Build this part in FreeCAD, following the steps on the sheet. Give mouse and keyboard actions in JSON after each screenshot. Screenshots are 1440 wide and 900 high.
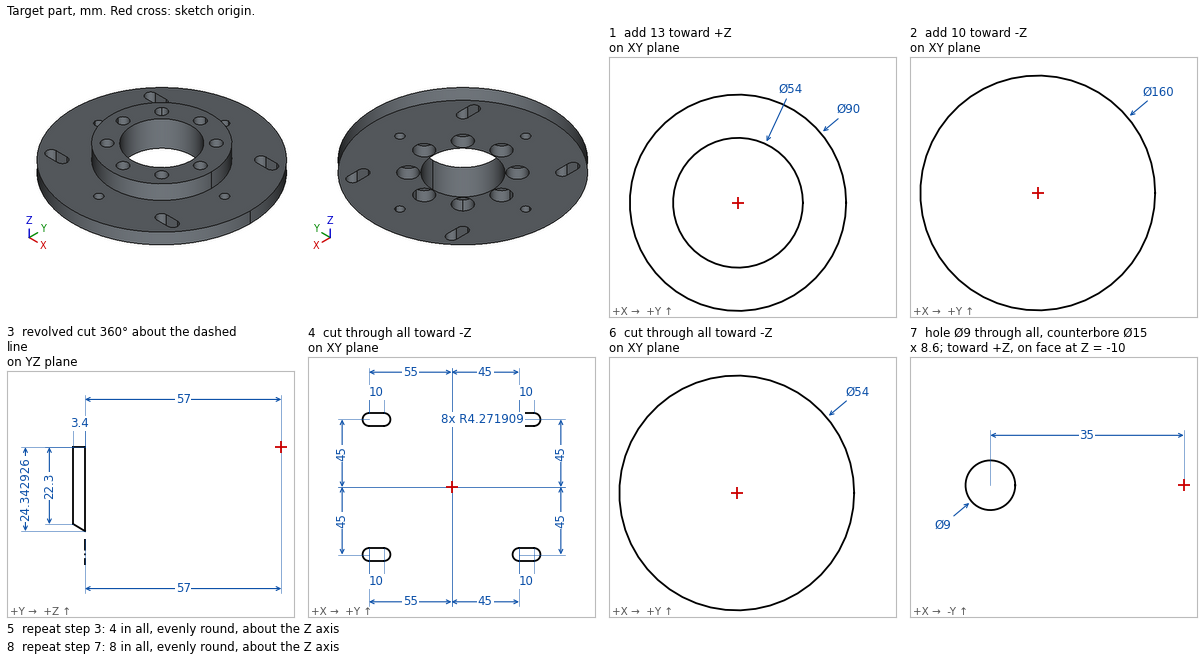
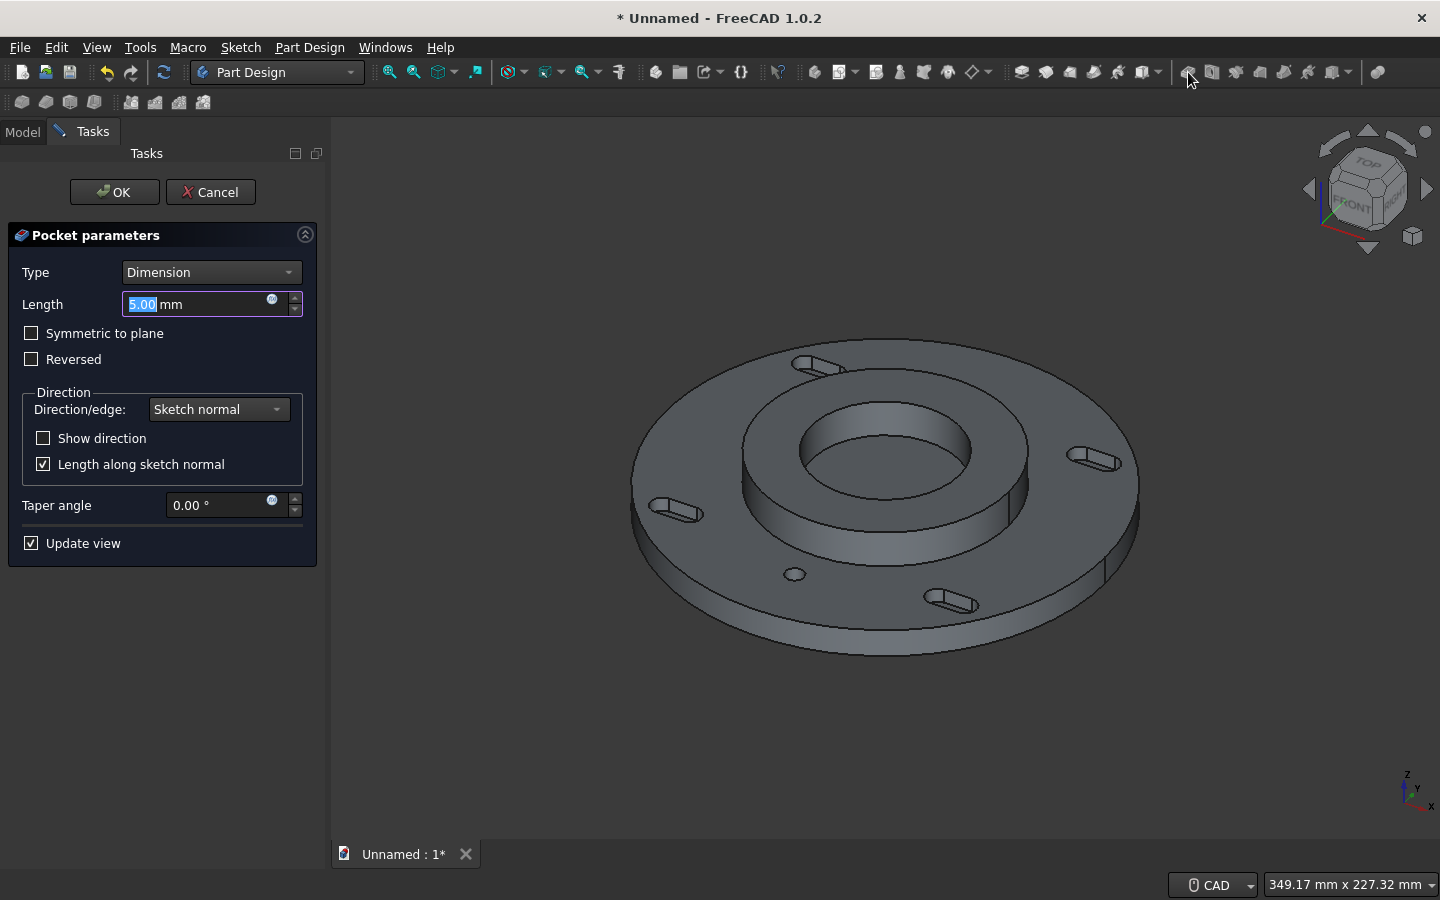
{"action": "left_click", "coordinate": [212, 272]}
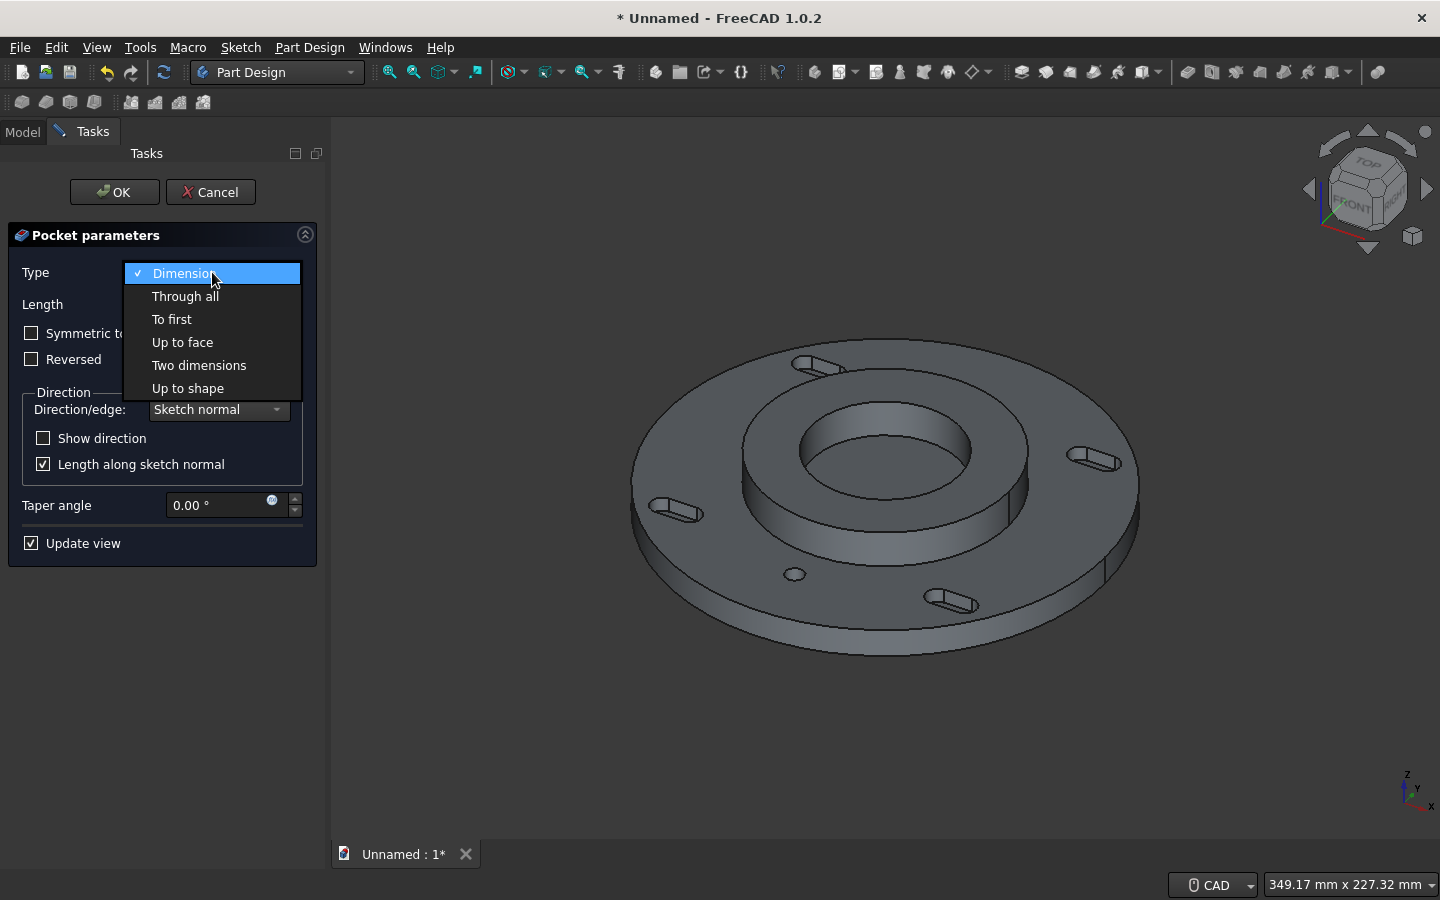
{"action": "left_click", "coordinate": [212, 296]}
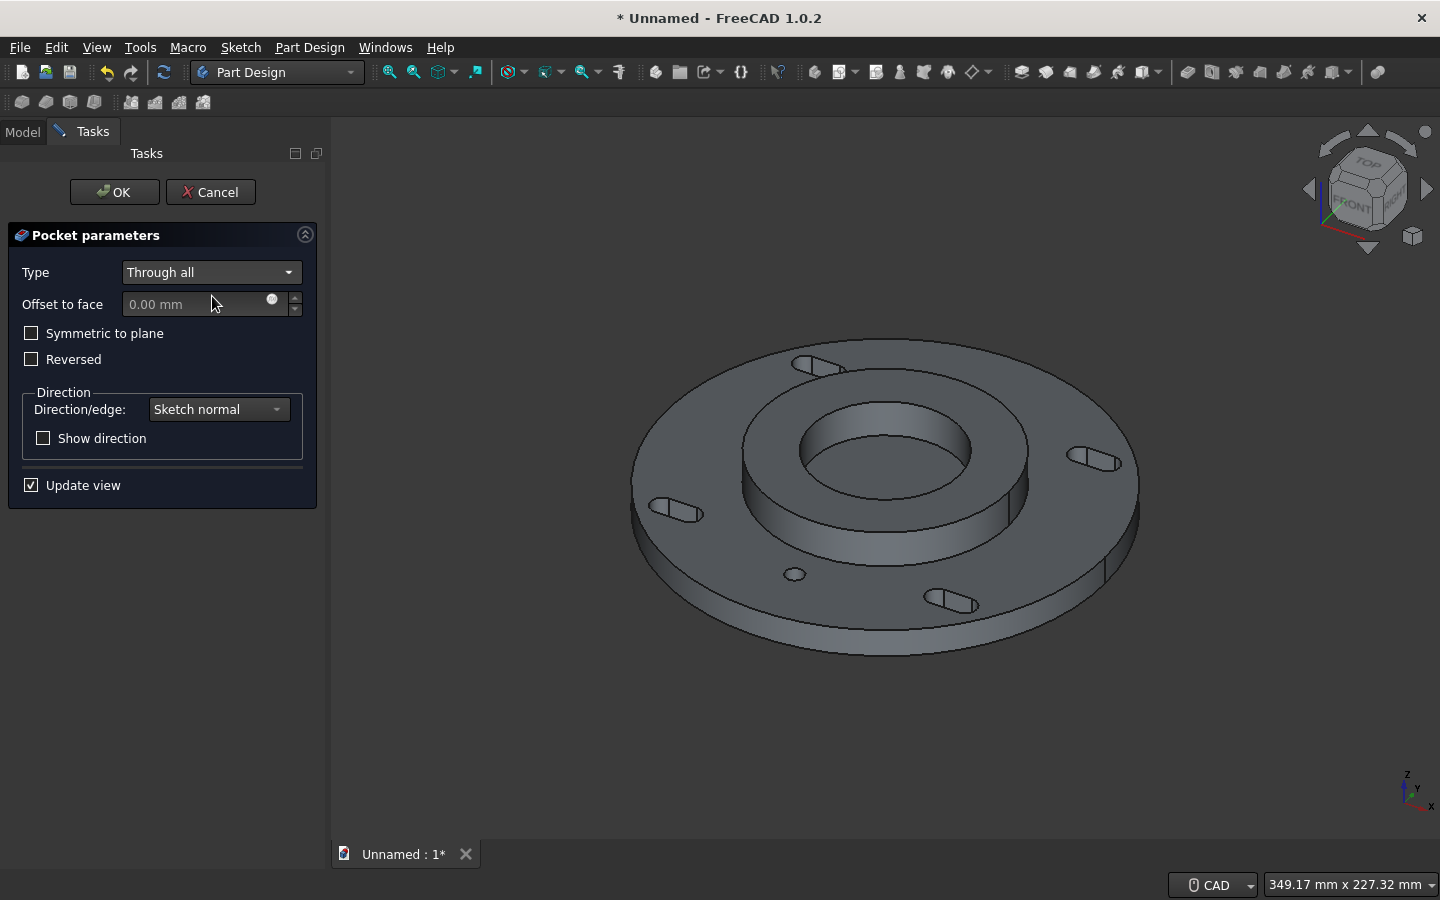
{"action": "left_click", "coordinate": [115, 192]}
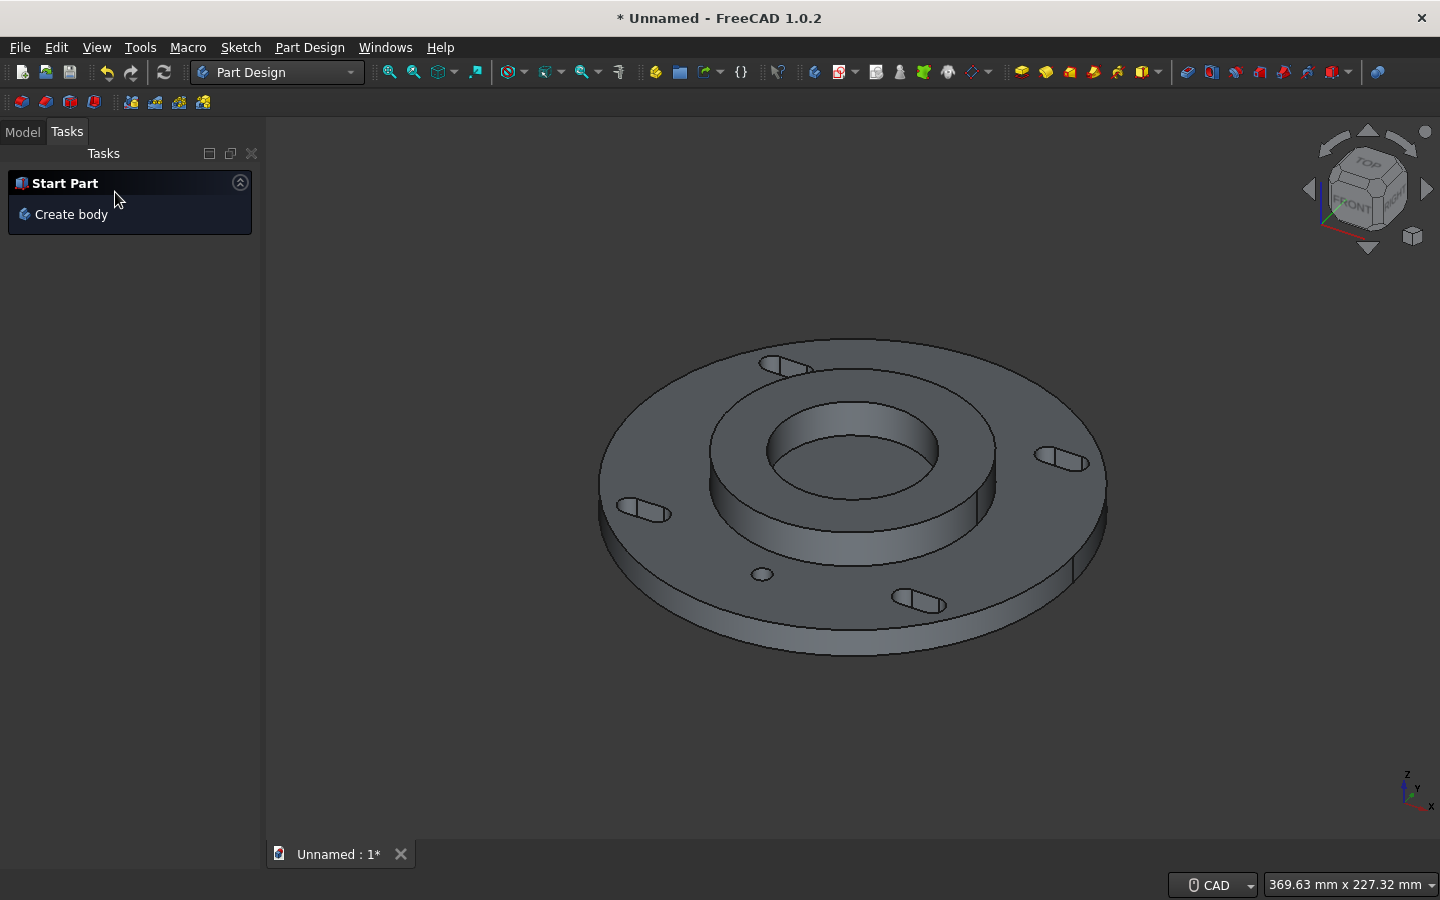
{"action": "left_click", "coordinate": [23, 131]}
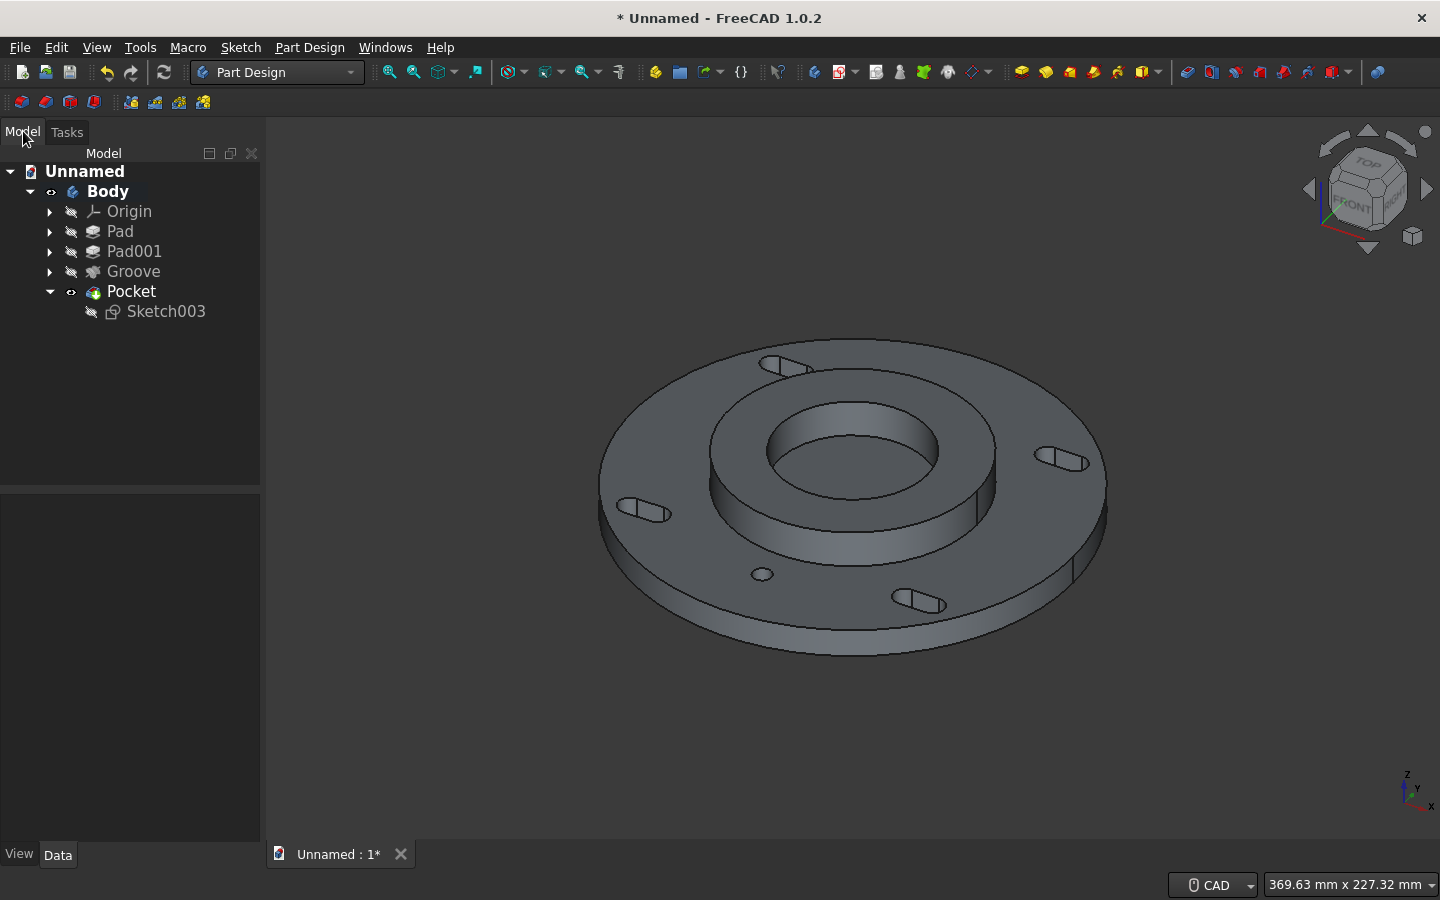
{"action": "left_click", "coordinate": [116, 272]}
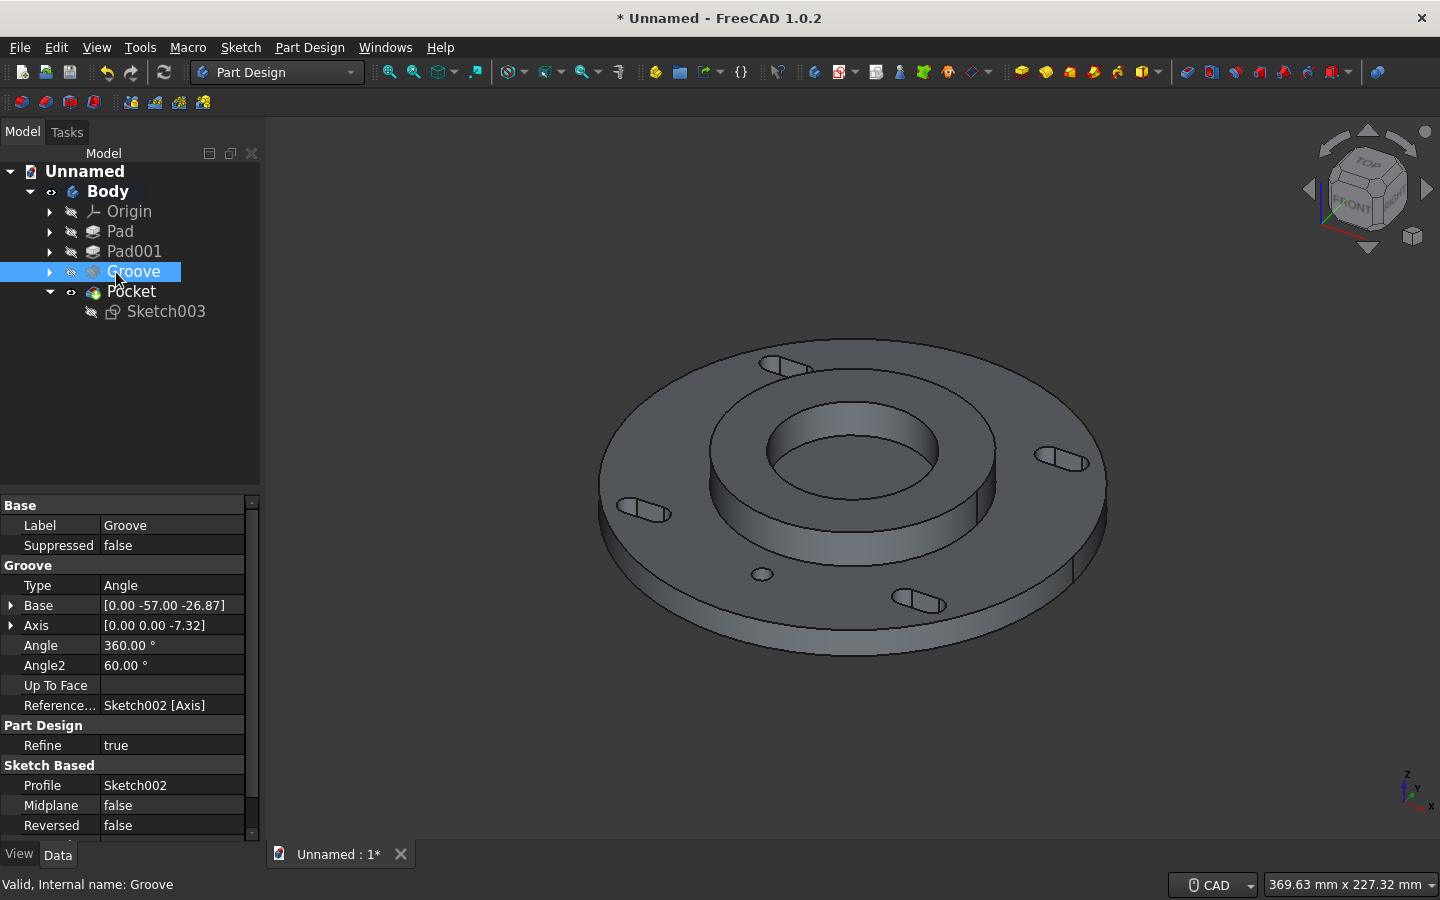
{"action": "left_click", "coordinate": [180, 102]}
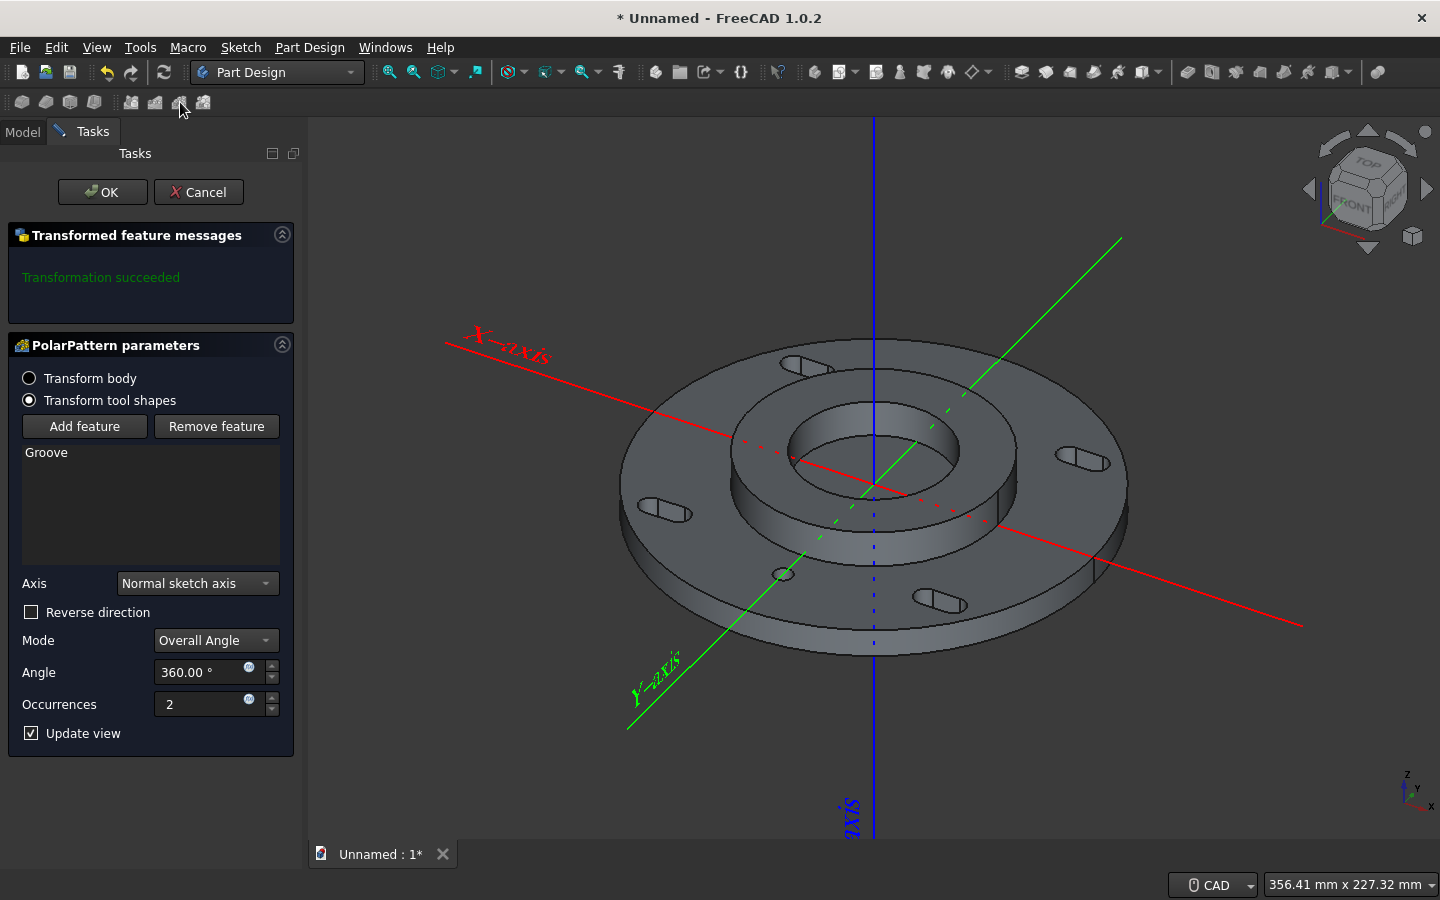
{"action": "left_click", "coordinate": [198, 584]}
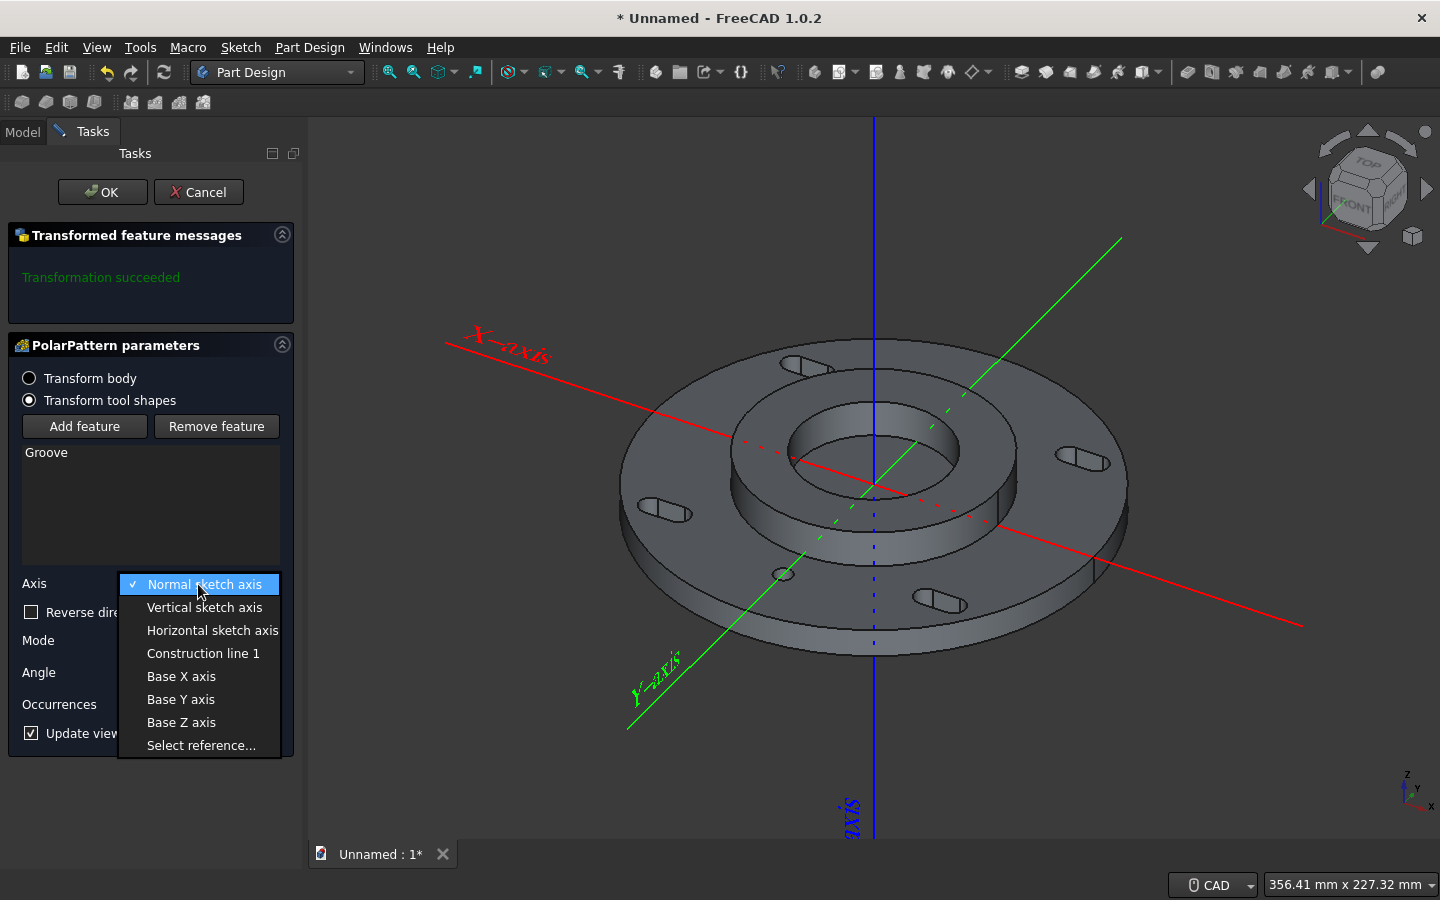
{"action": "left_click", "coordinate": [198, 722]}